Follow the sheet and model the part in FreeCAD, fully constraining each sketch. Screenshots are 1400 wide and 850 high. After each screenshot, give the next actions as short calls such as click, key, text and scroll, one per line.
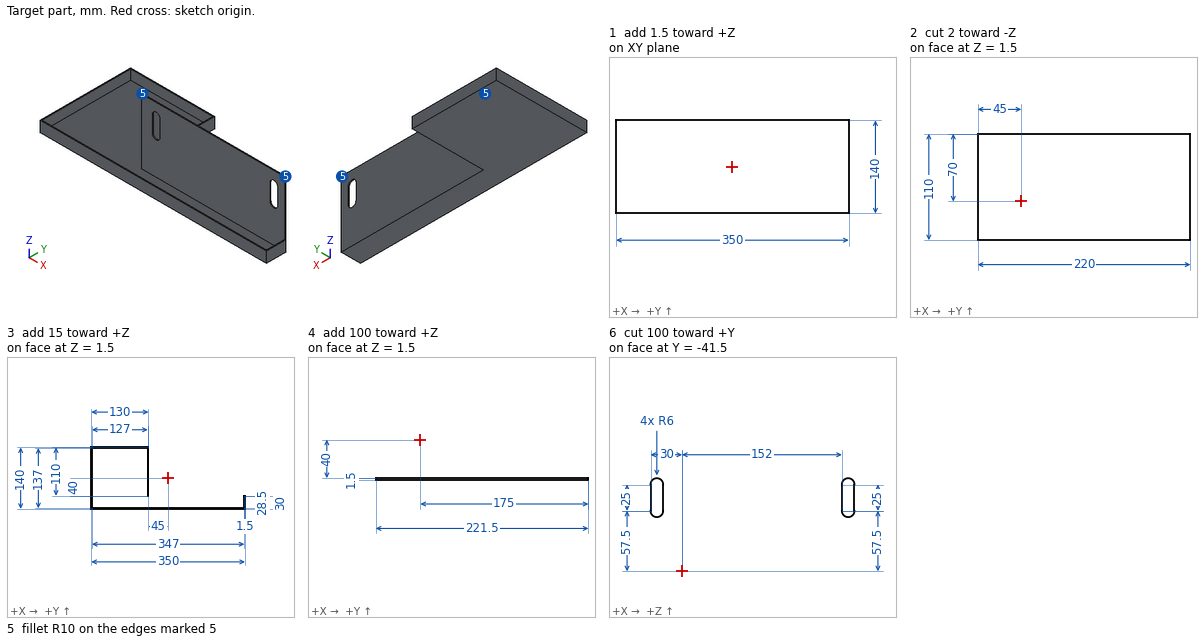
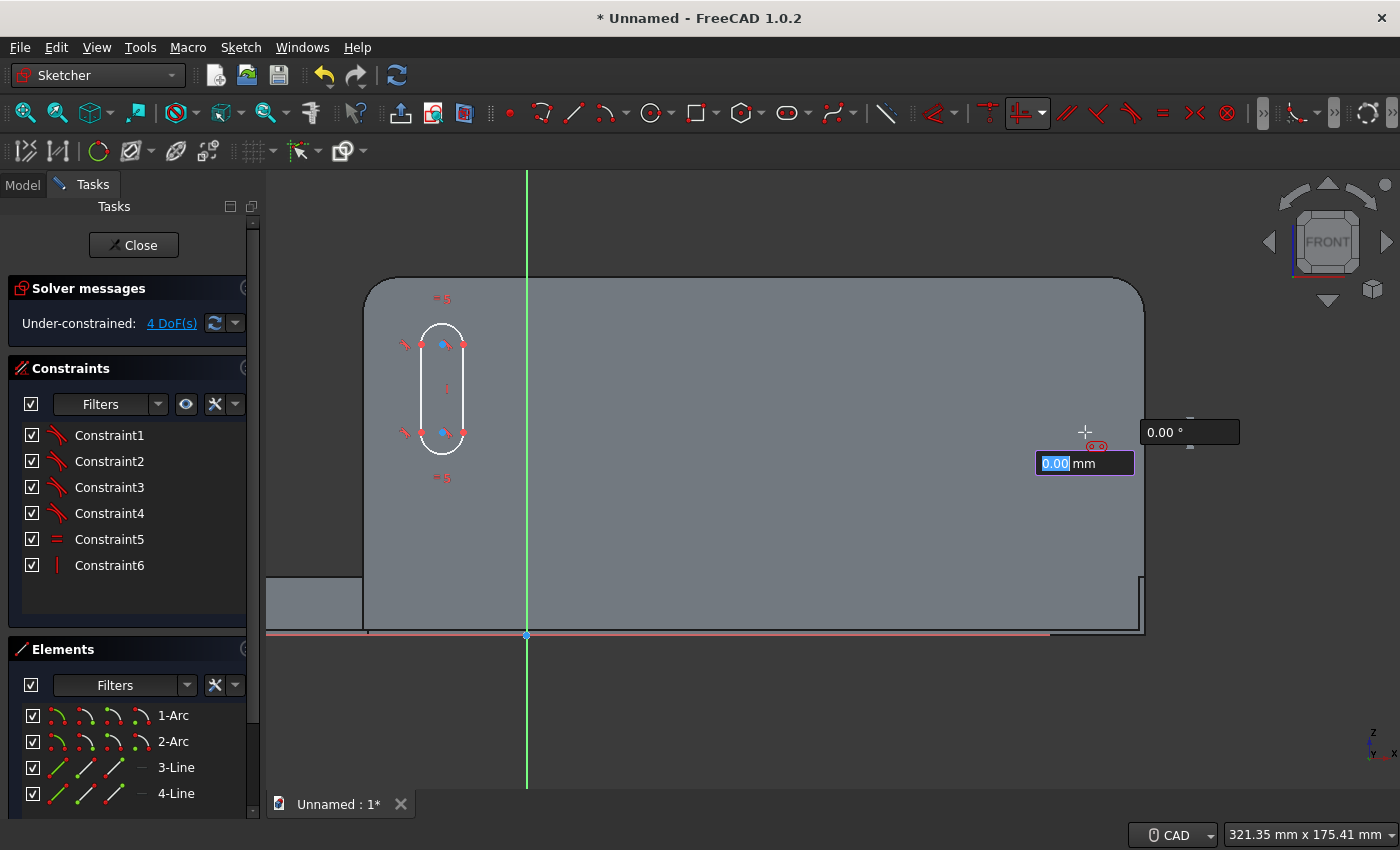
click(1085, 344)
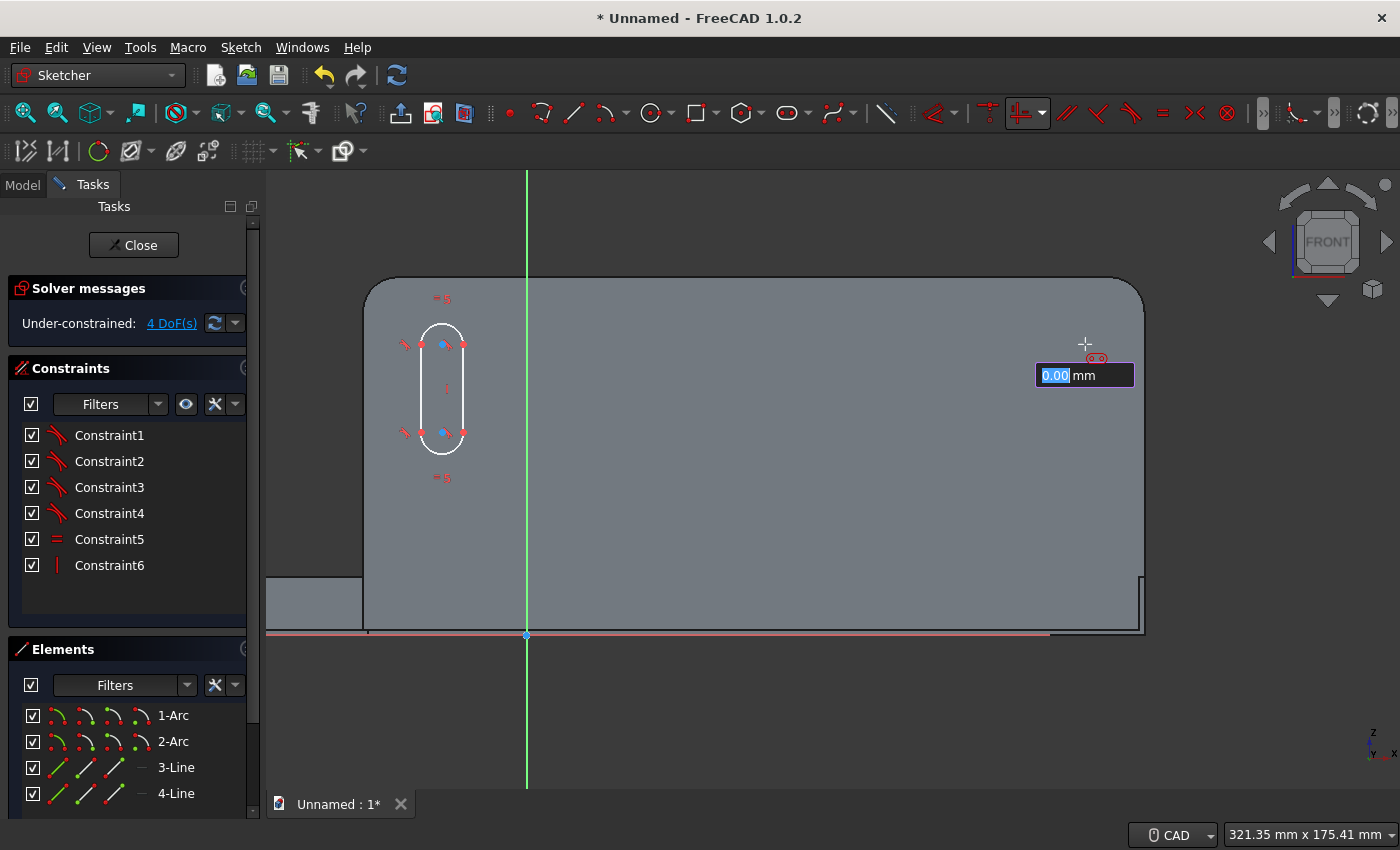
click(1106, 388)
key(Escape)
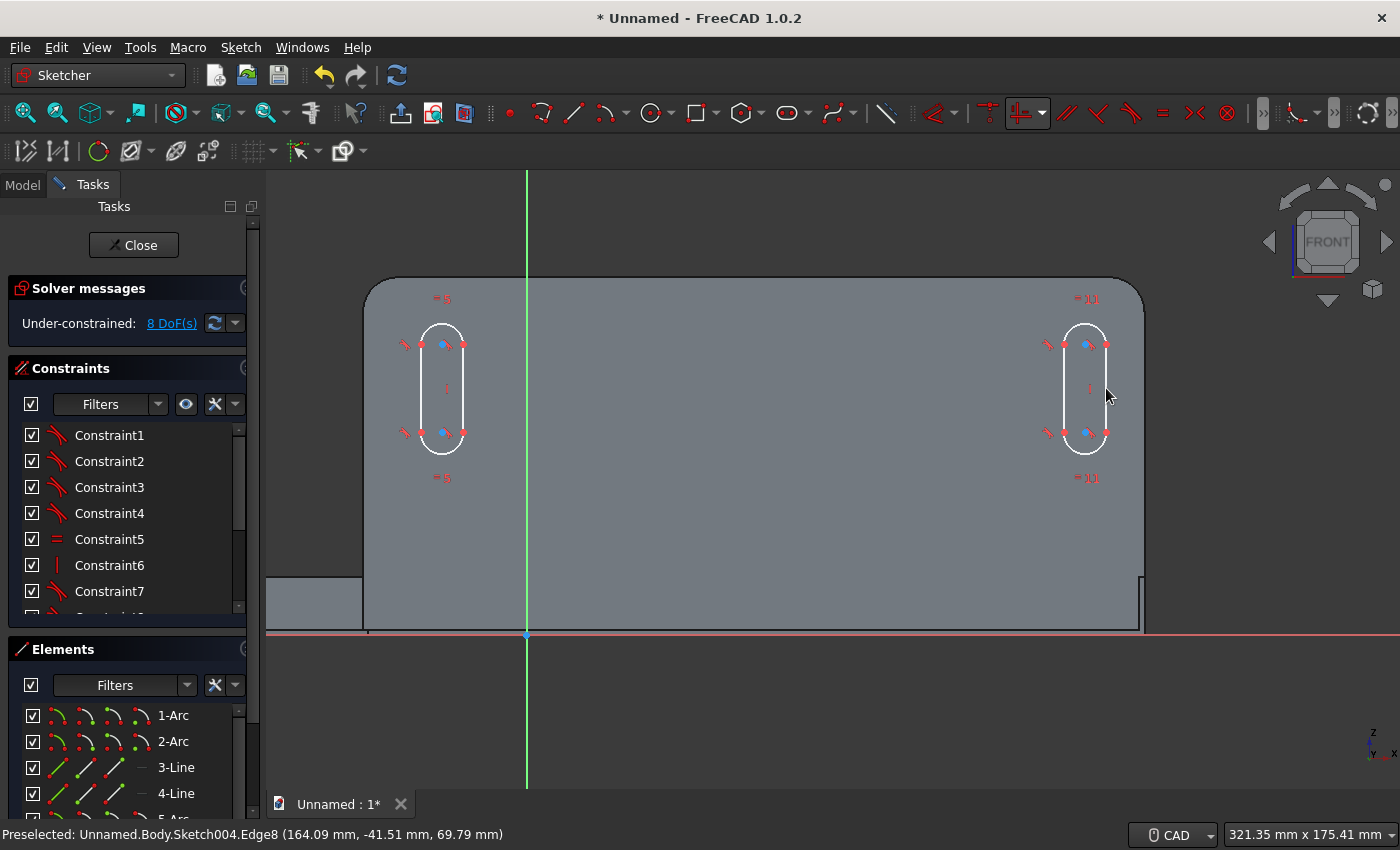
click(430, 450)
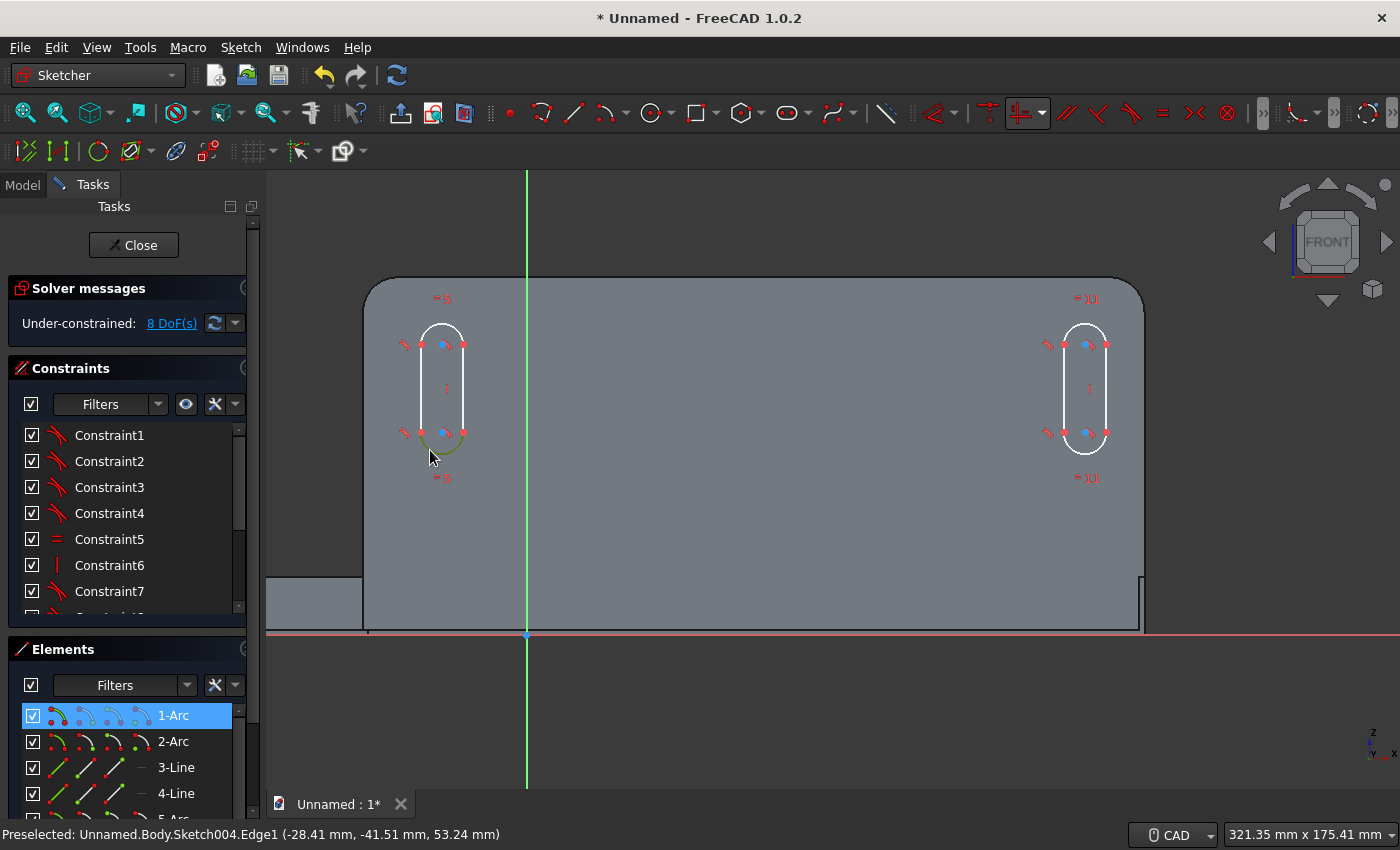
click(1073, 450)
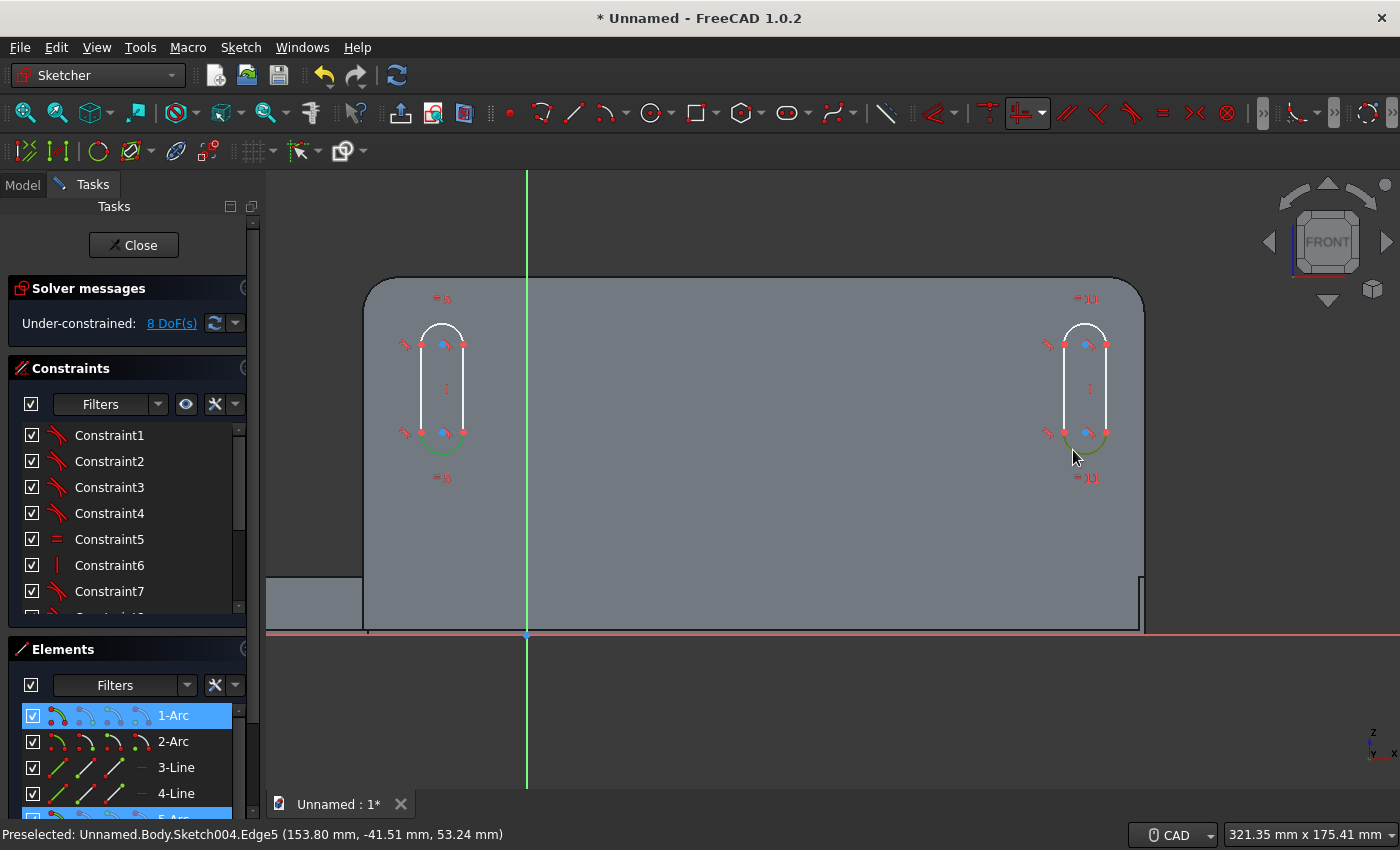
key(e)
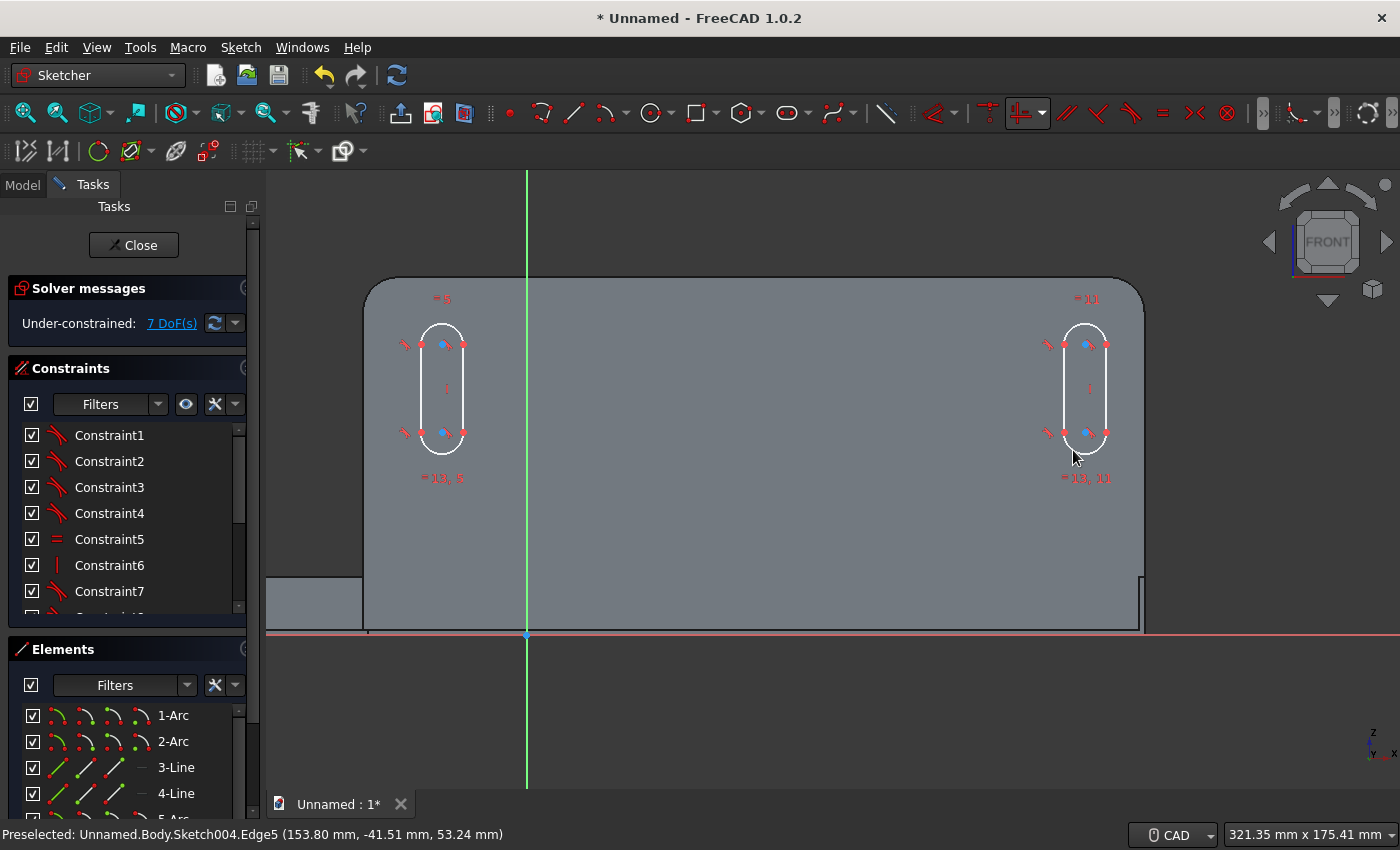
key(d)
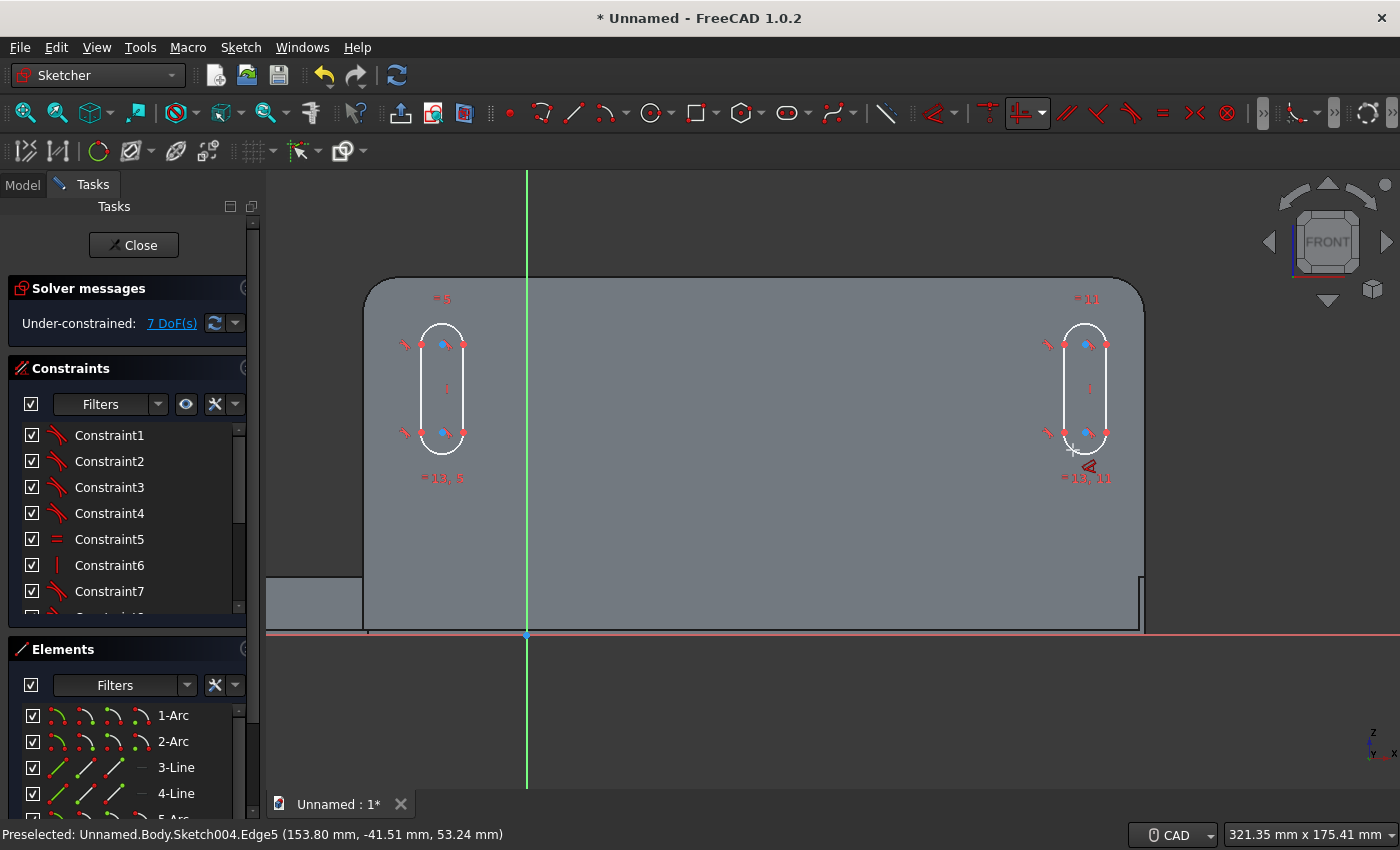
scroll(430, 450, up, 4)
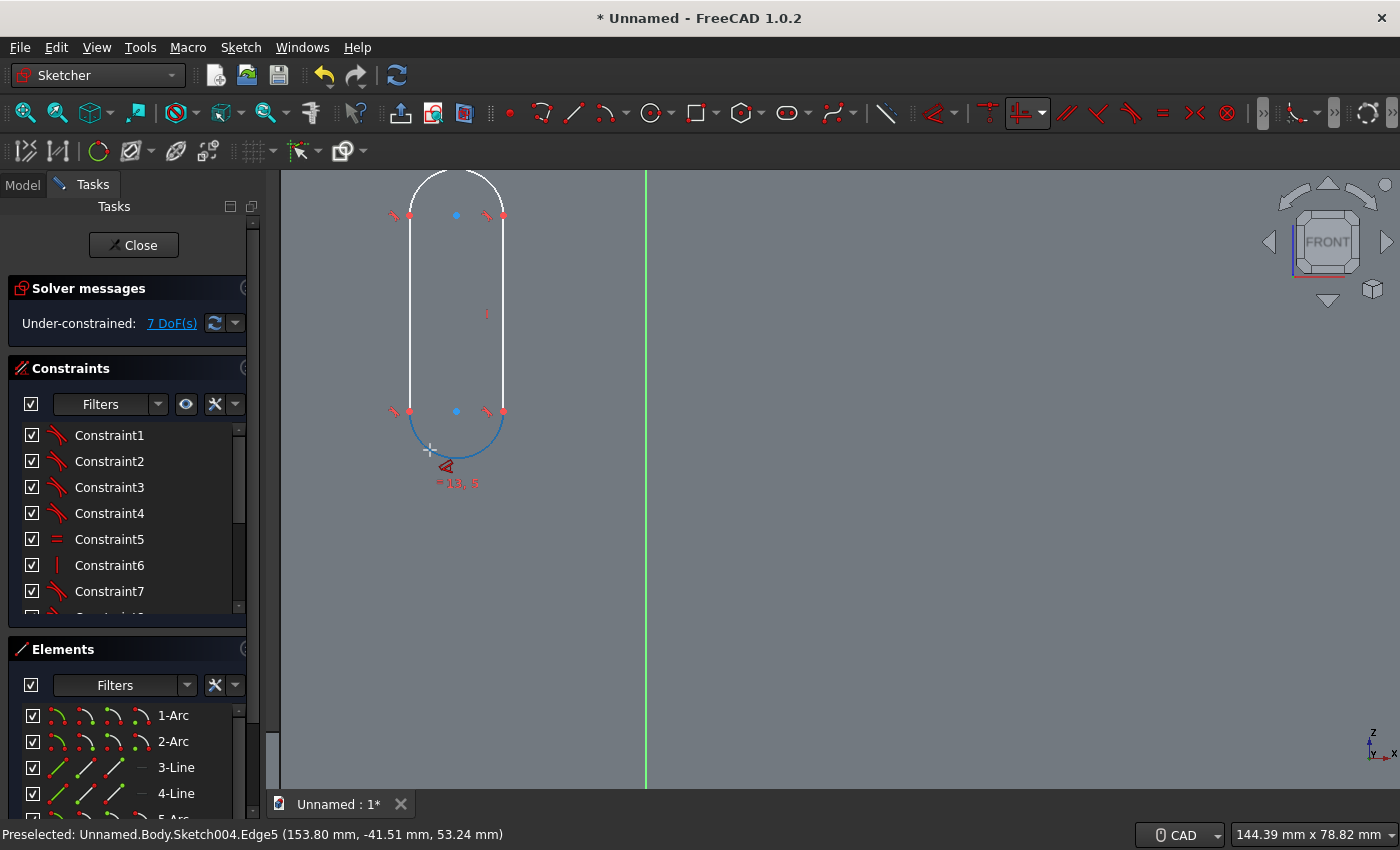
click(429, 449)
click(410, 475)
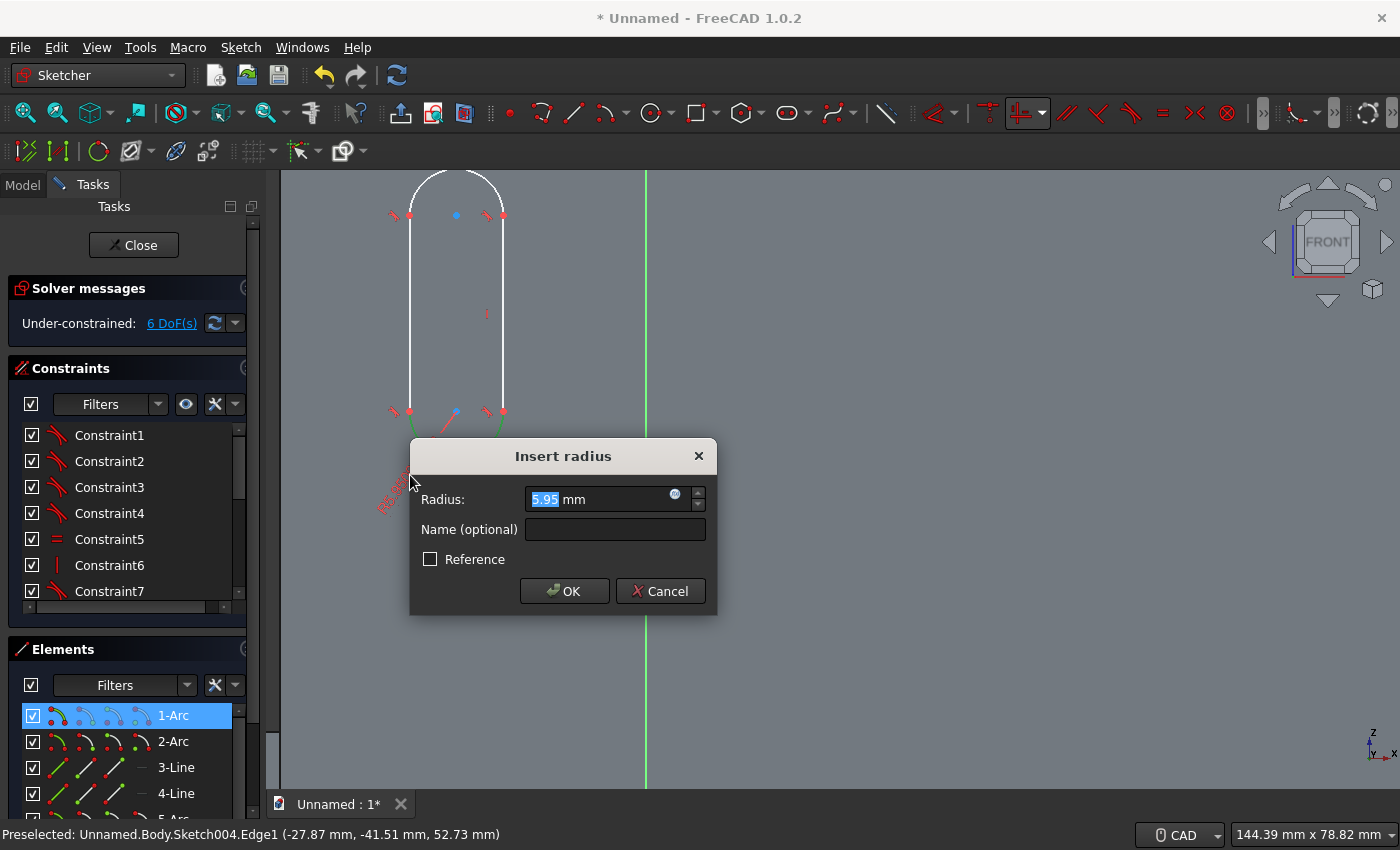
text(6)
key(Return)